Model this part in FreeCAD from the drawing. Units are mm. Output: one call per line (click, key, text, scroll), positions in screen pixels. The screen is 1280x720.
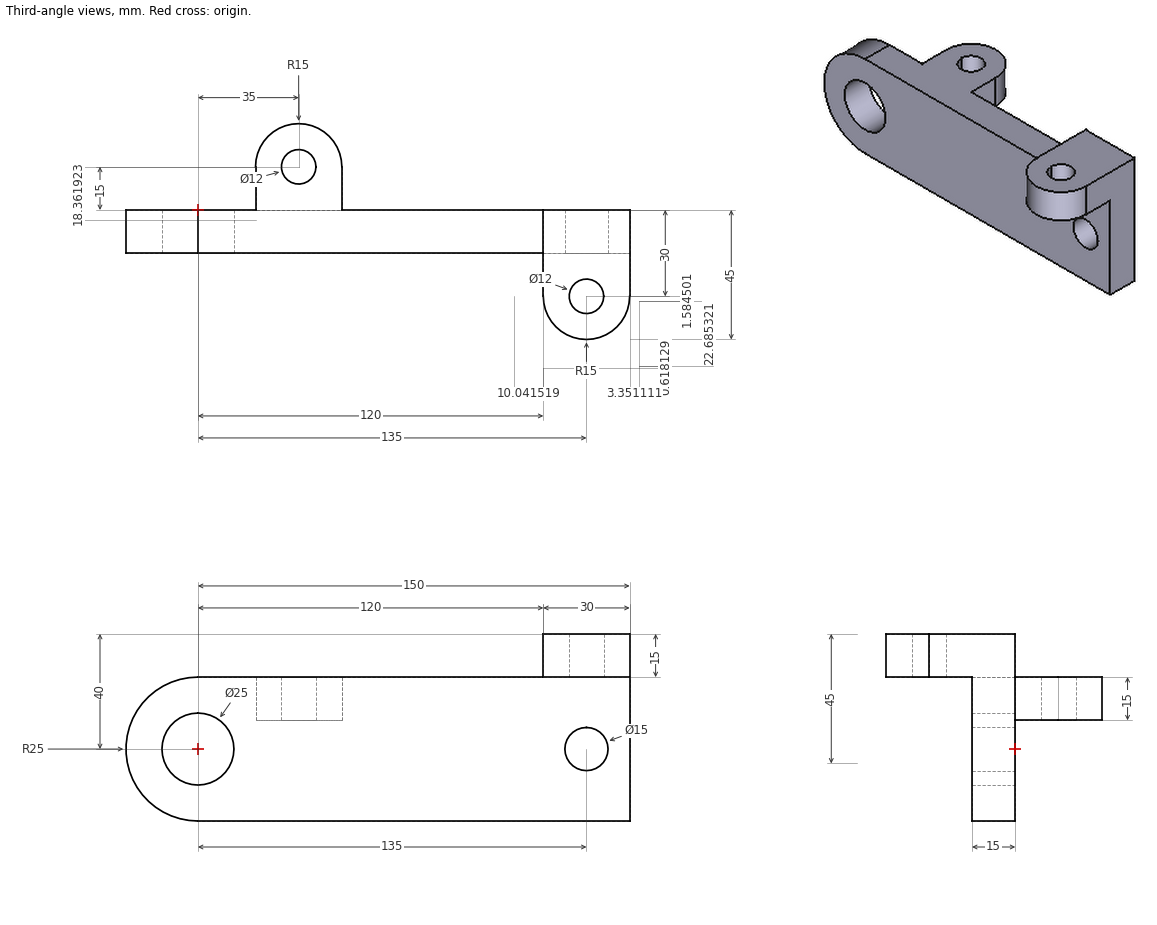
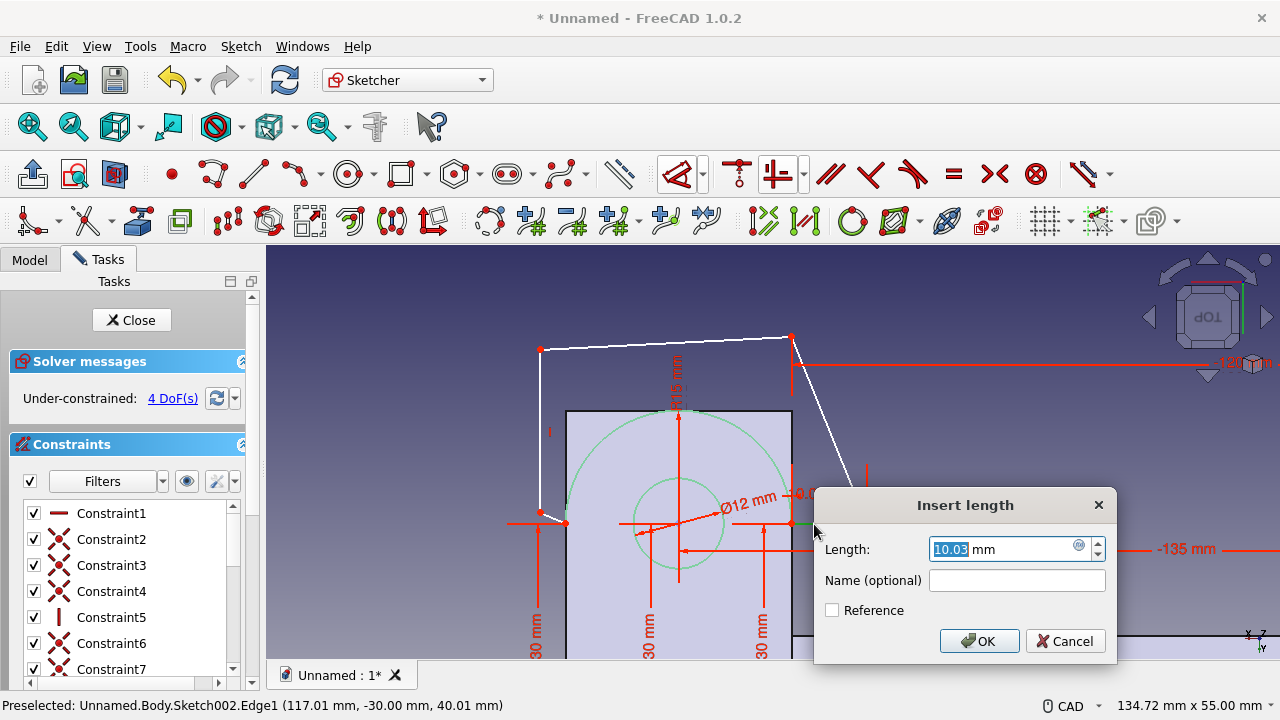
text(10.041519)
key(Return)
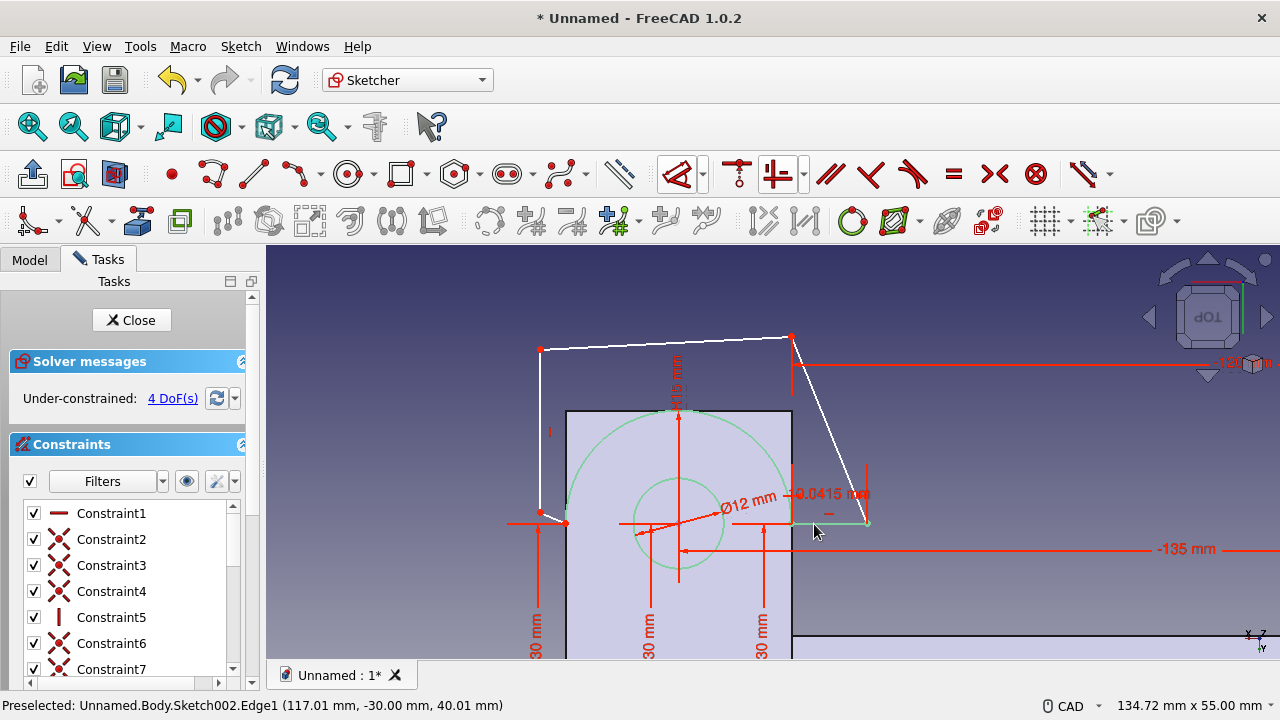
click(540, 399)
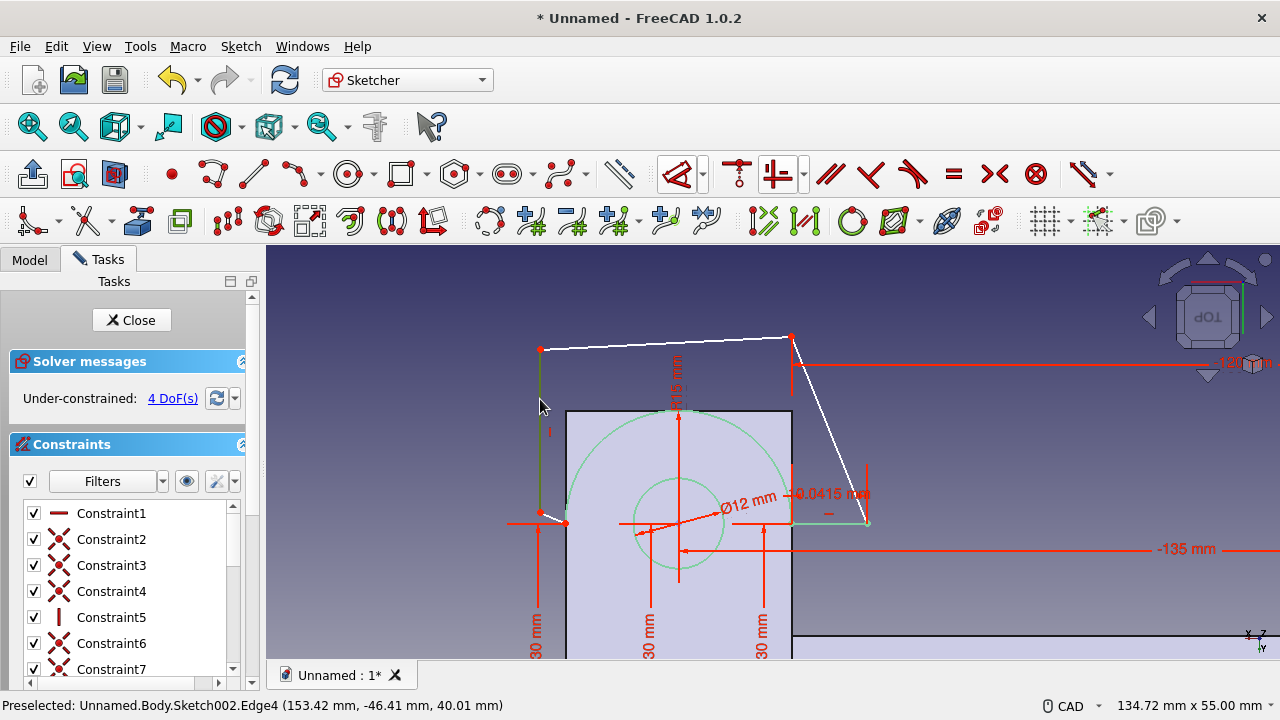
click(702, 174)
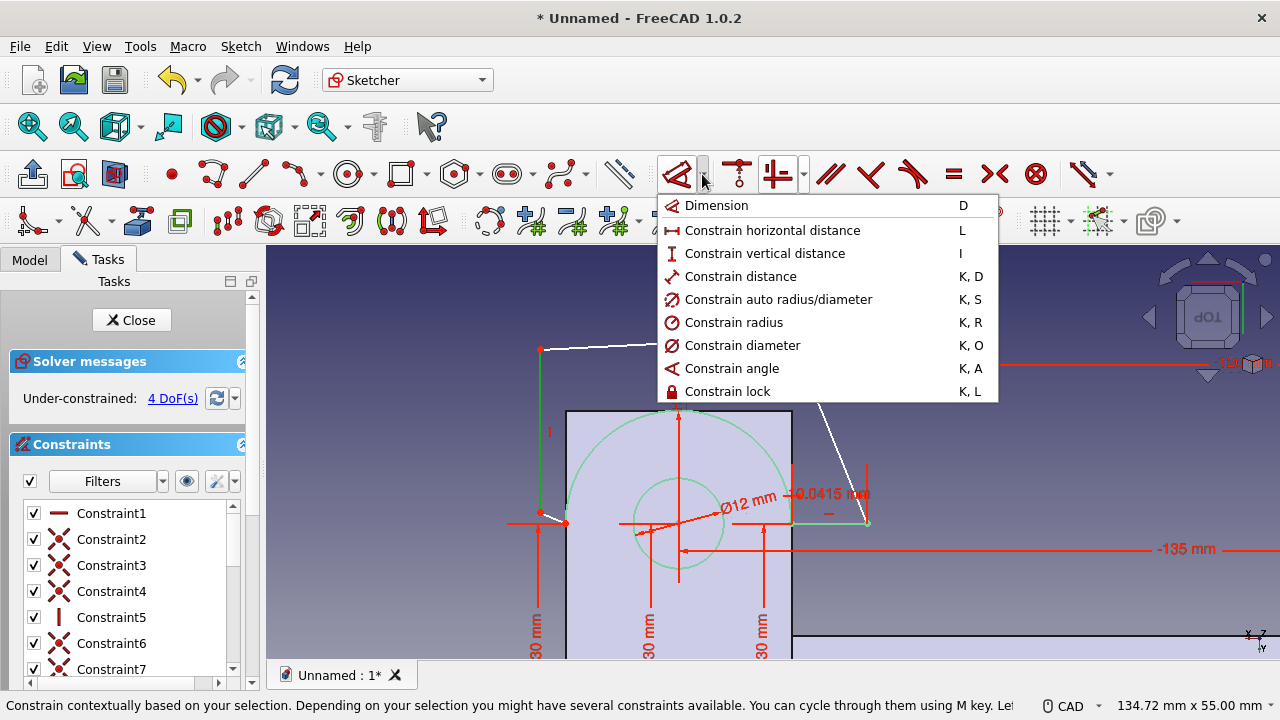
click(828, 254)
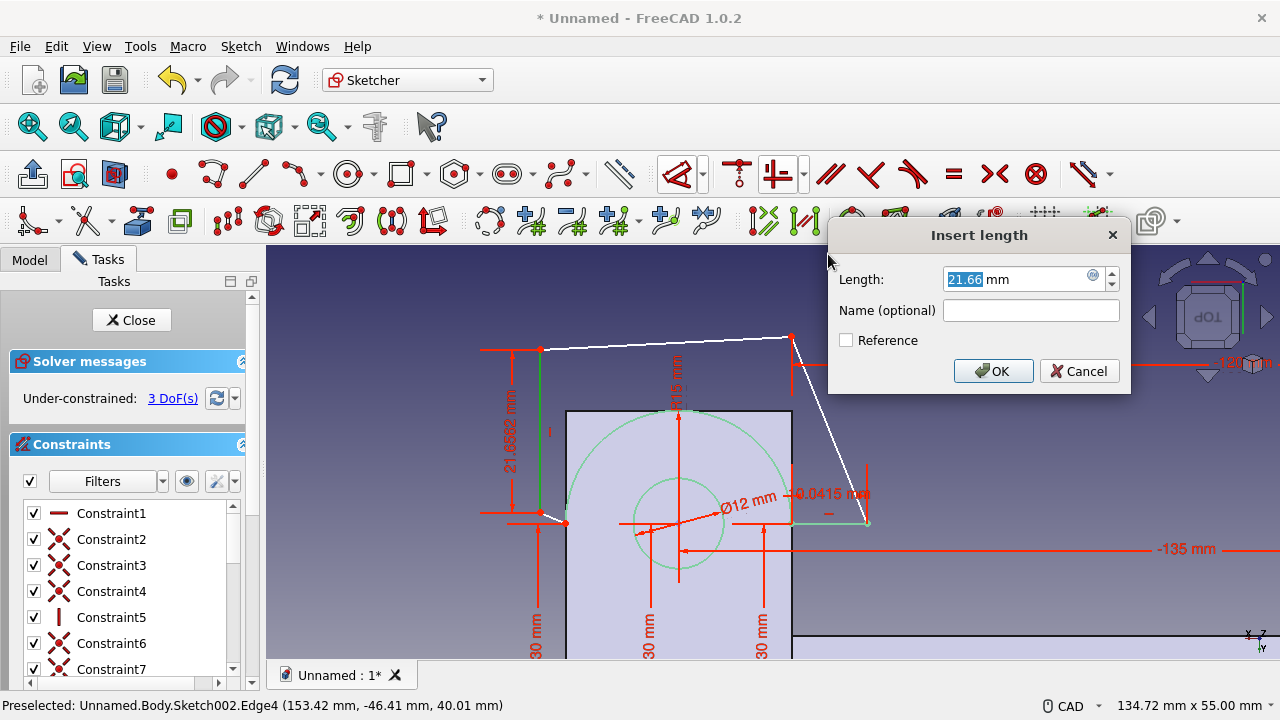
text(22.685321)
key(Return)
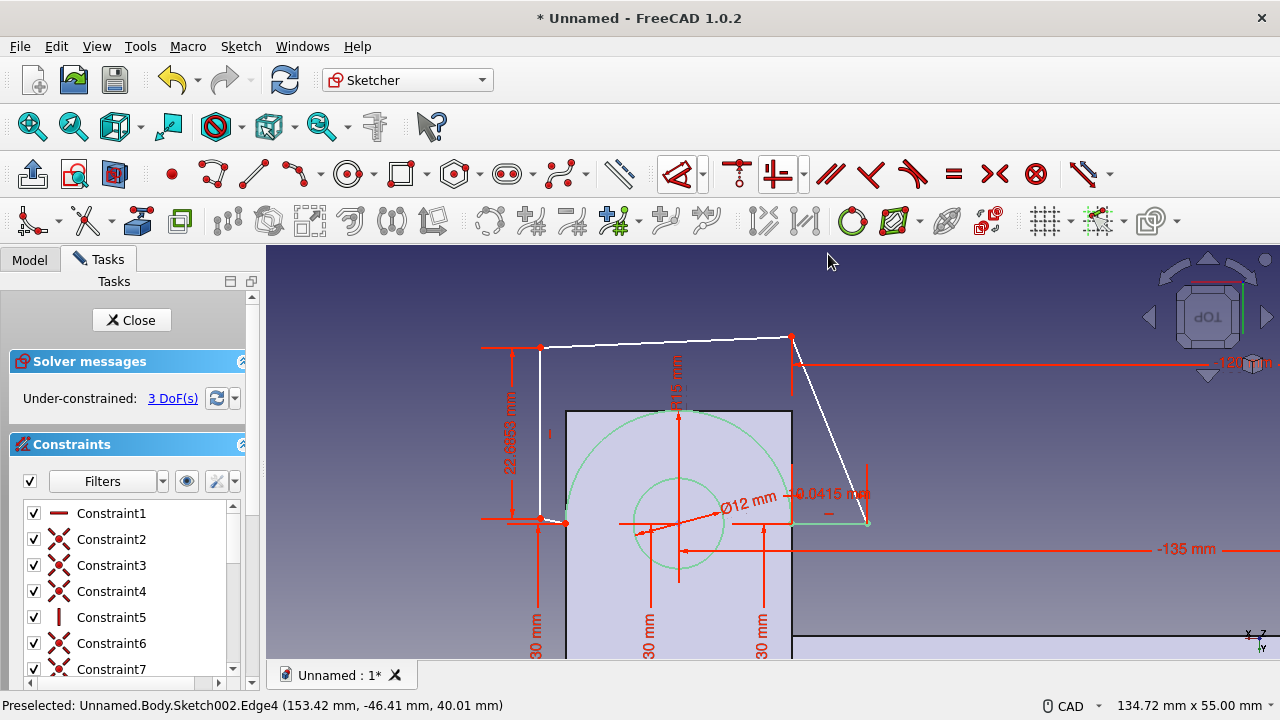
scroll(716, 340, up, 11)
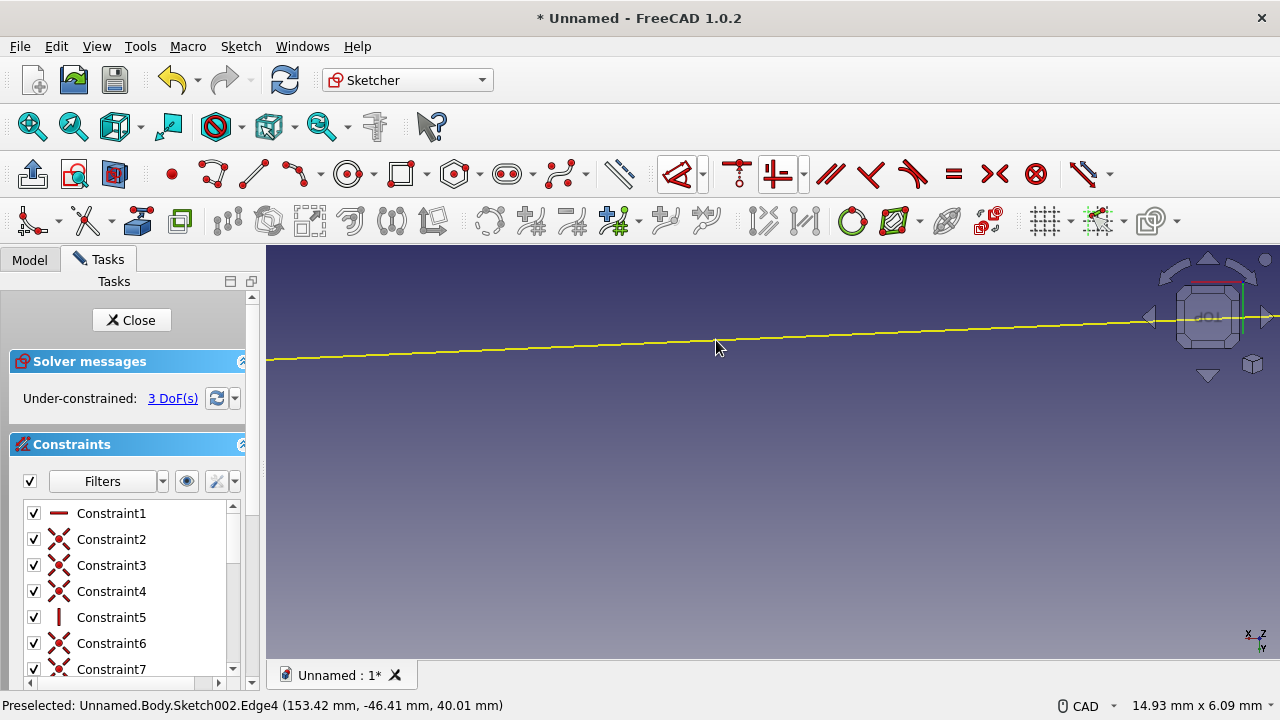
click(713, 341)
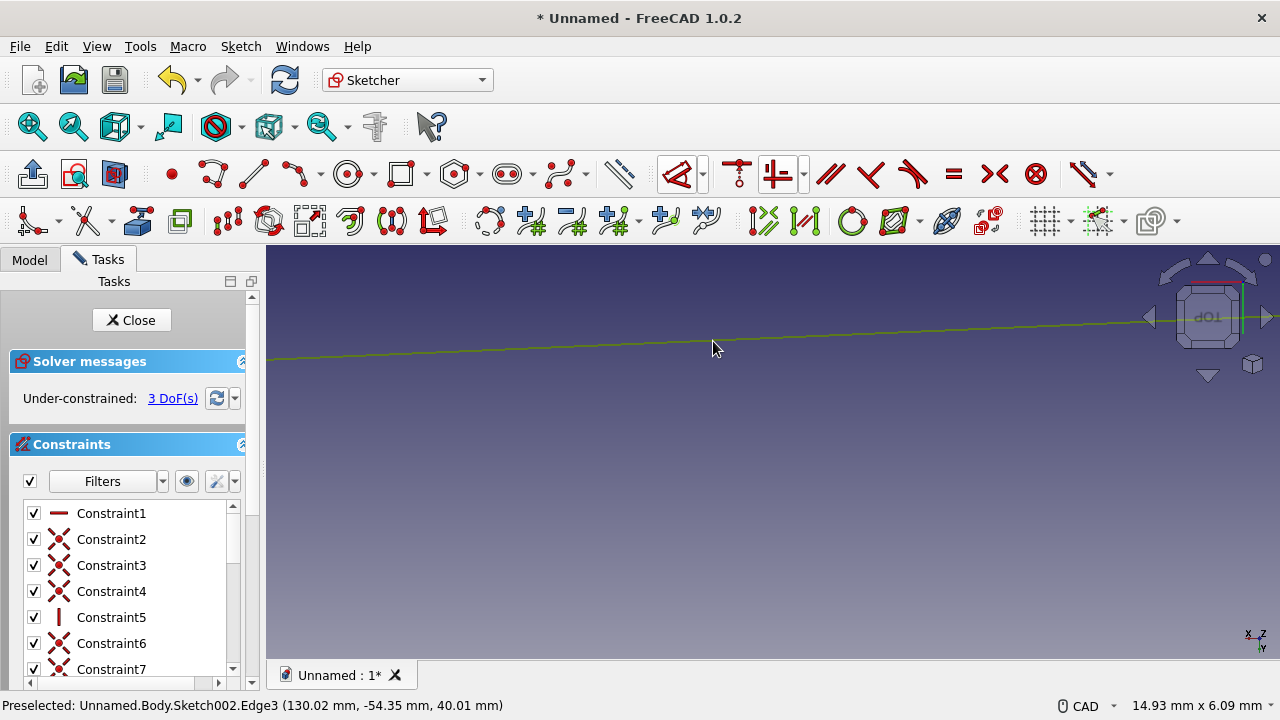
key(i)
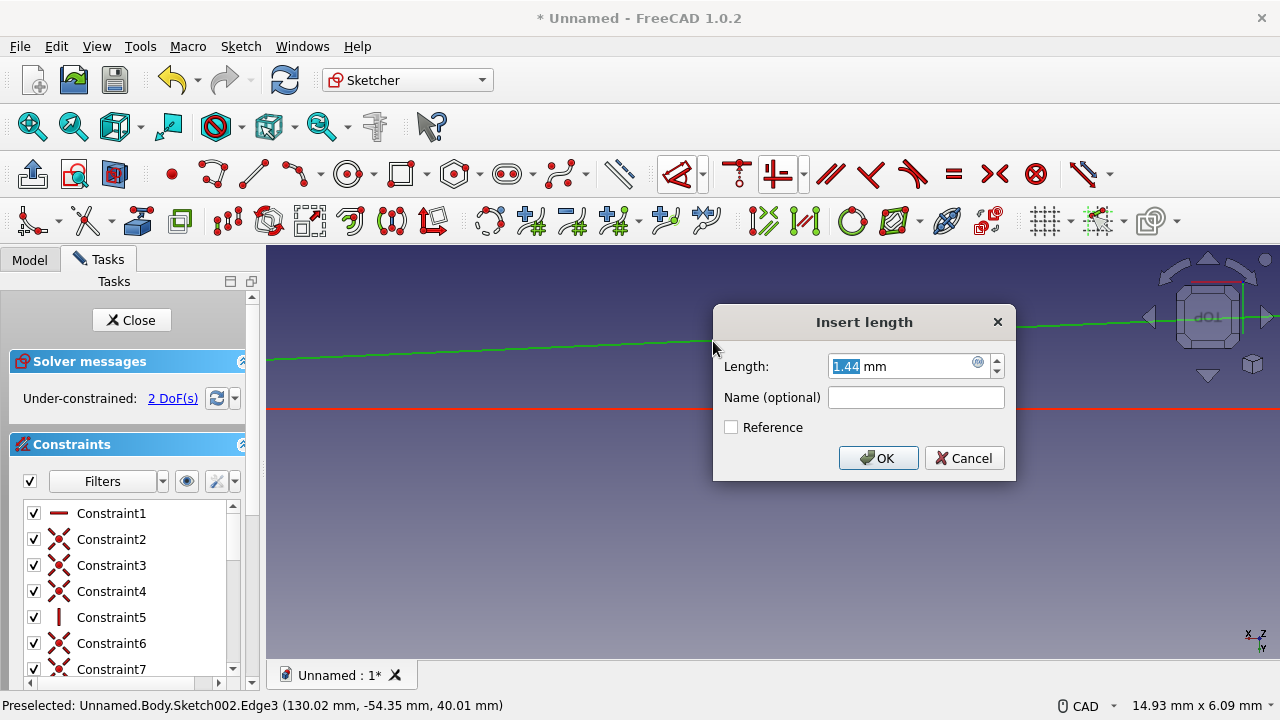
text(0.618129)
key(Return)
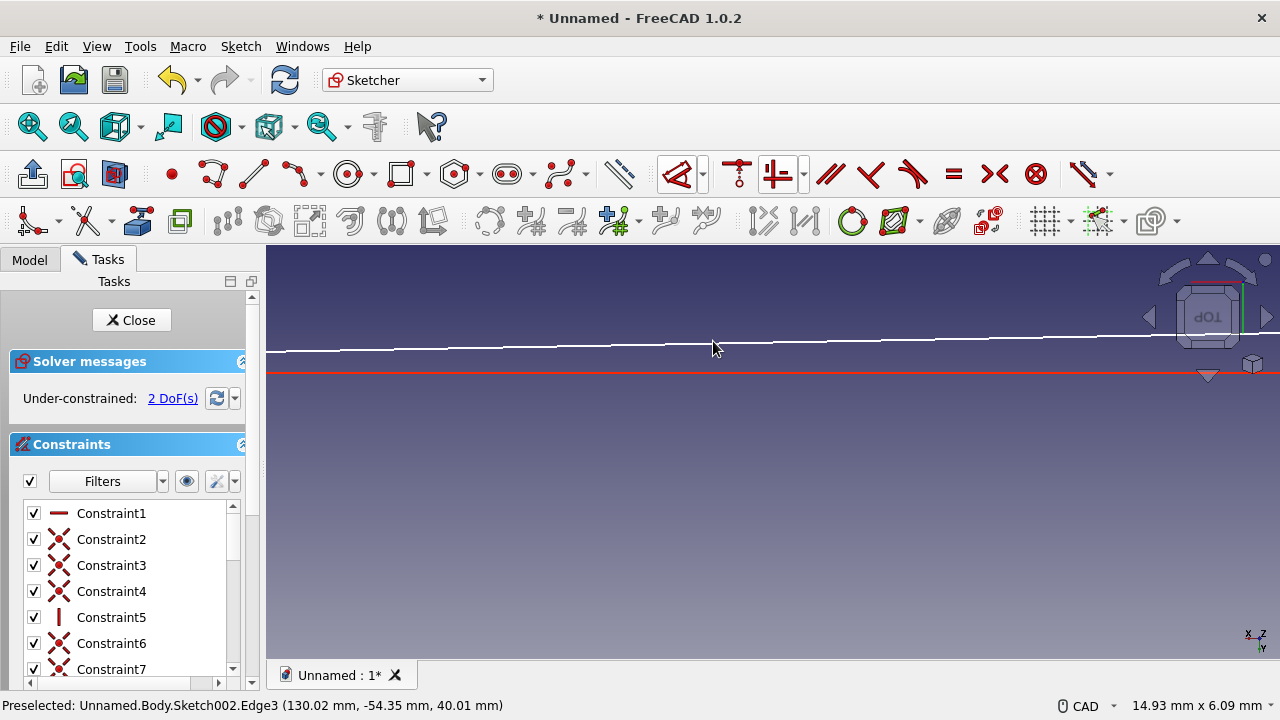
scroll(717, 340, down, 11)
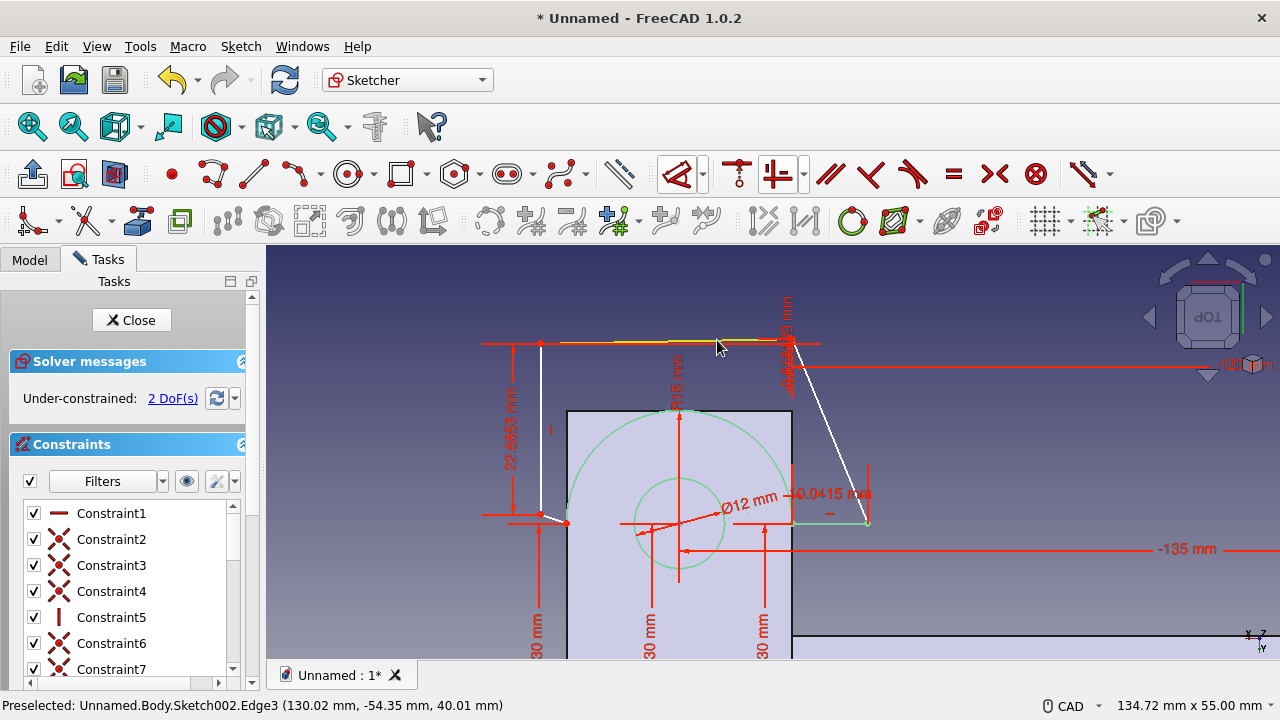
scroll(549, 517, up, 3)